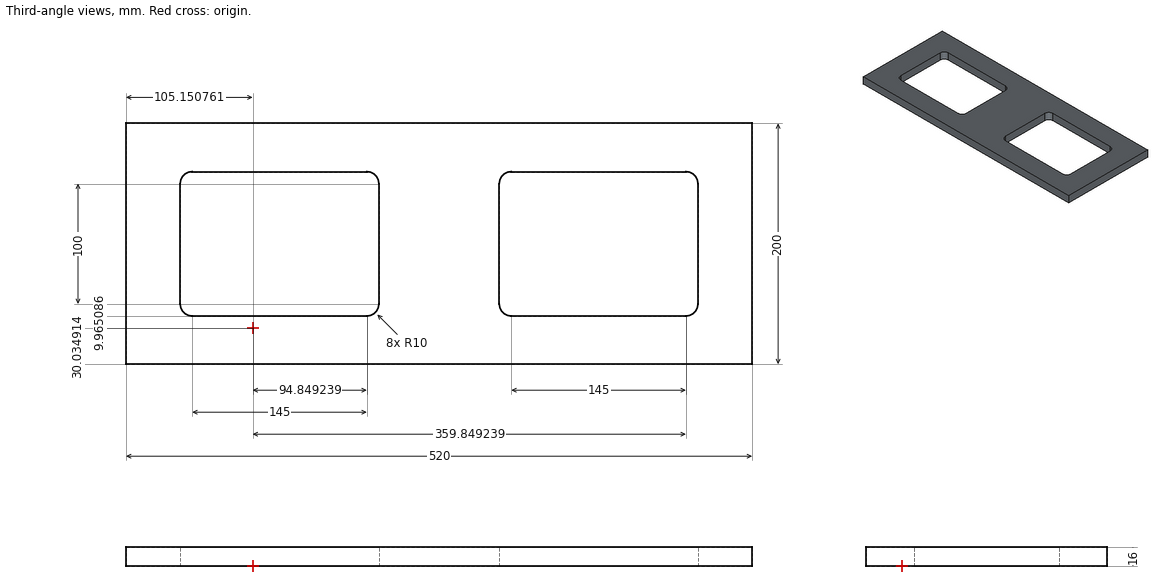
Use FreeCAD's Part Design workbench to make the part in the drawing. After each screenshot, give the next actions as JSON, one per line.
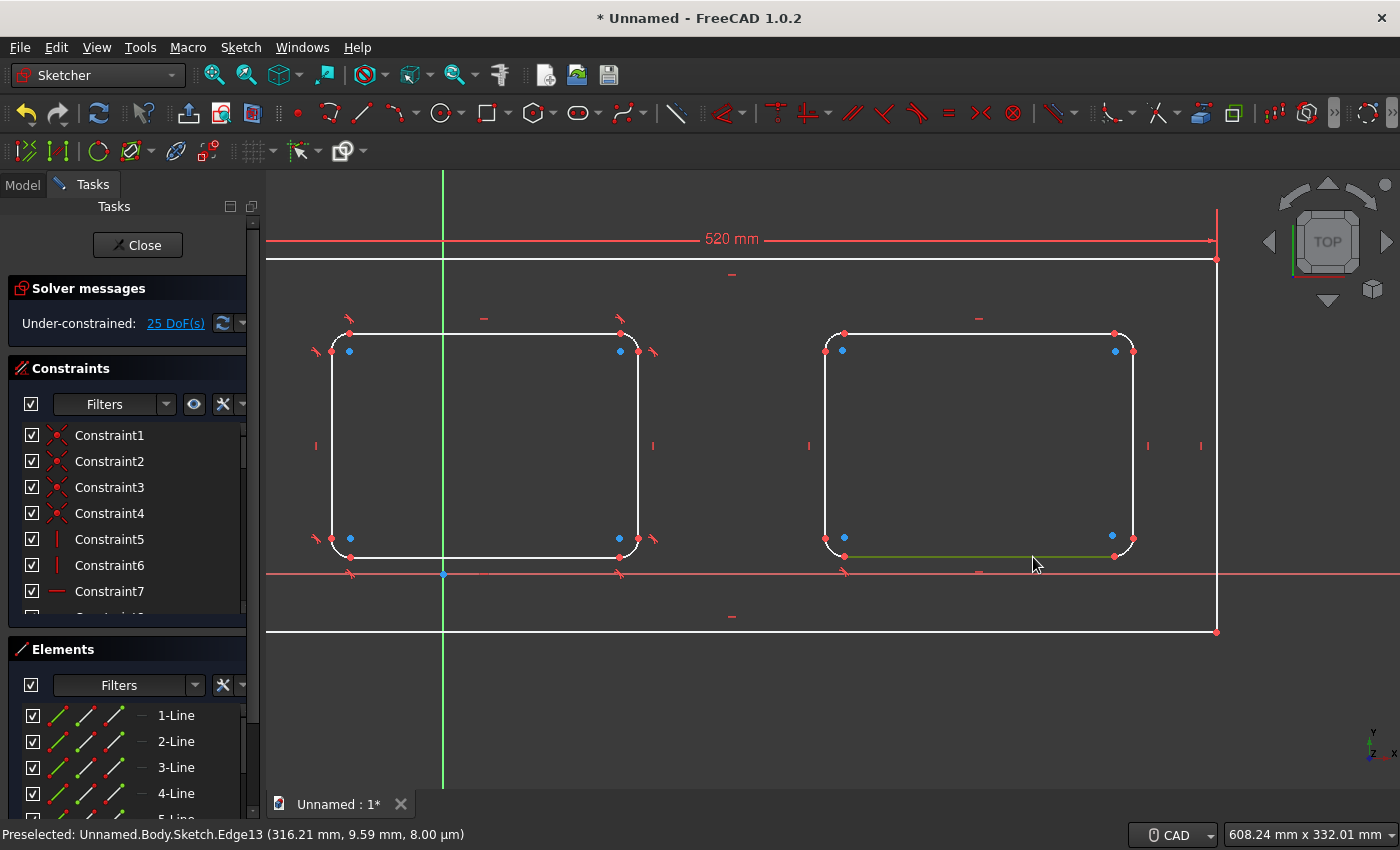
{"action": "left_click", "coordinate": [1127, 551]}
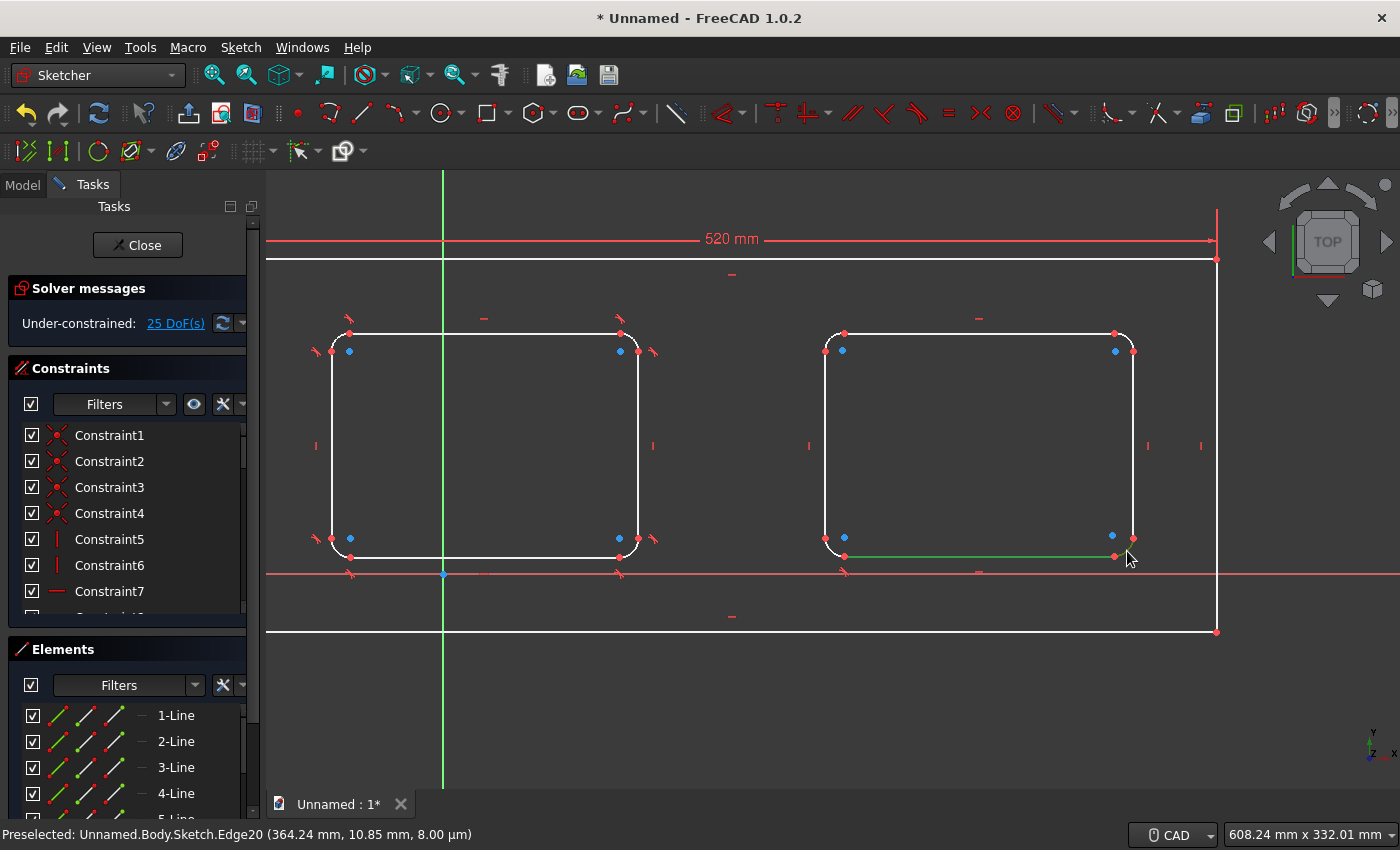
{"action": "key", "text": "t"}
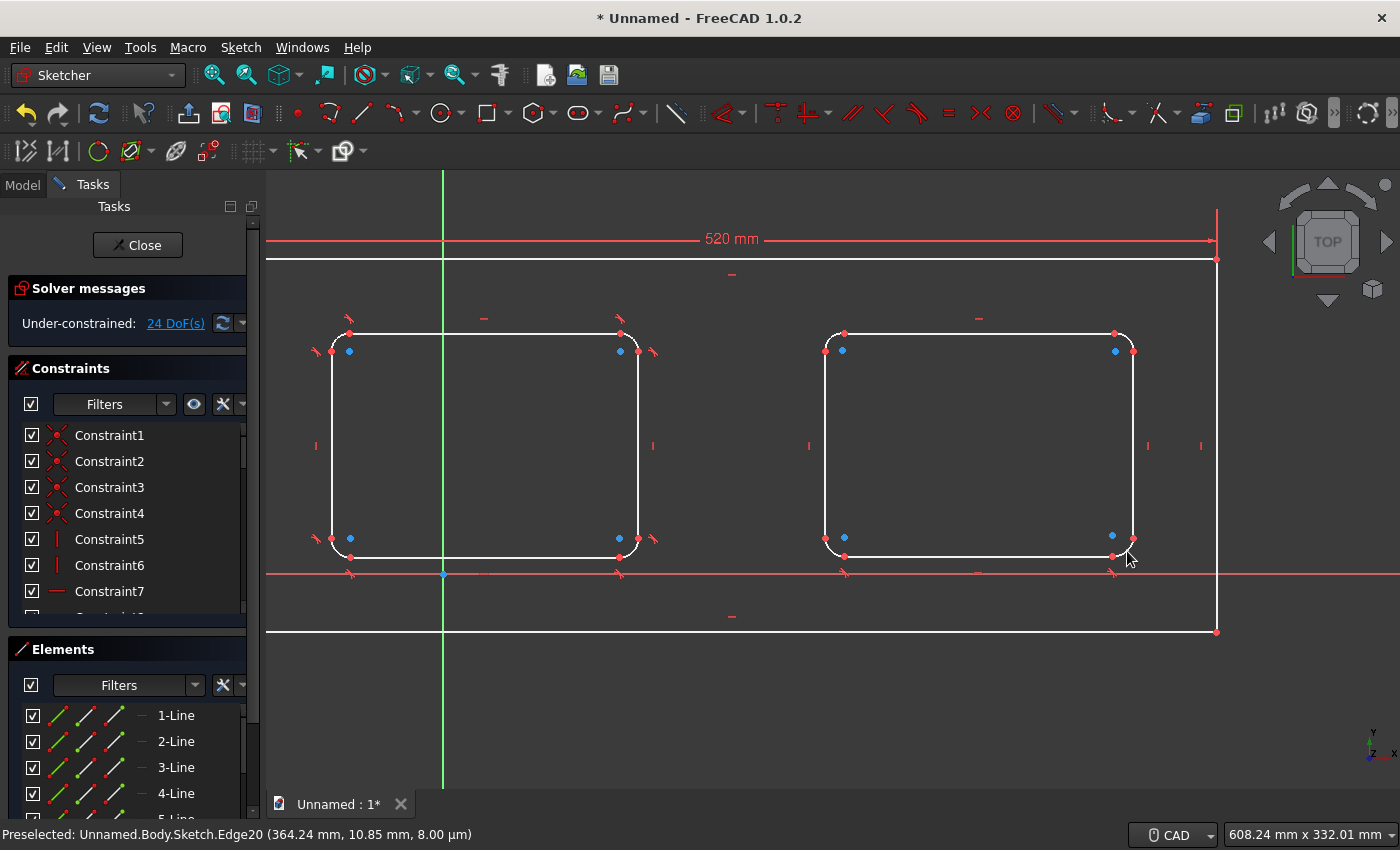
{"action": "left_click", "coordinate": [825, 482]}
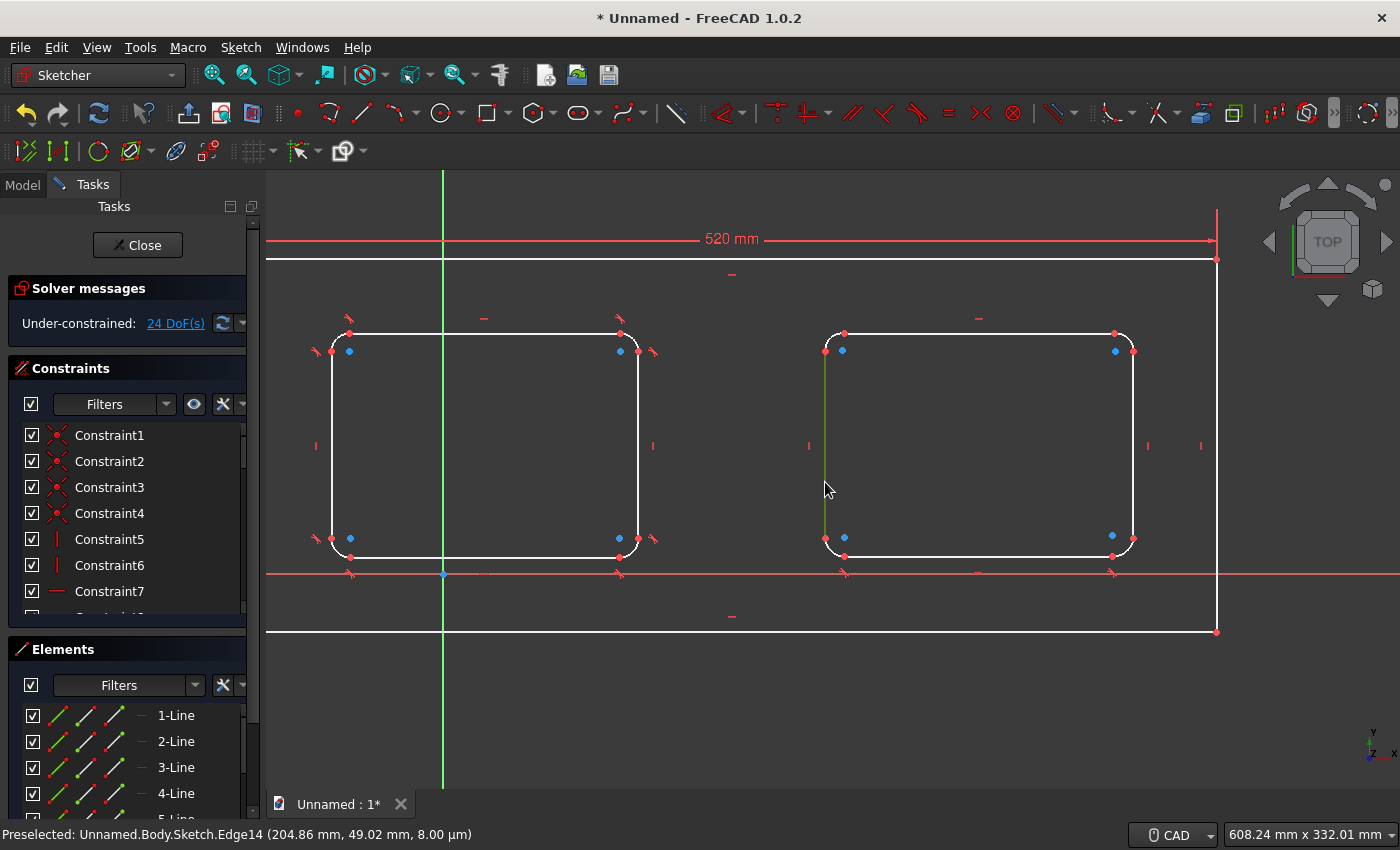
{"action": "left_click", "coordinate": [831, 551]}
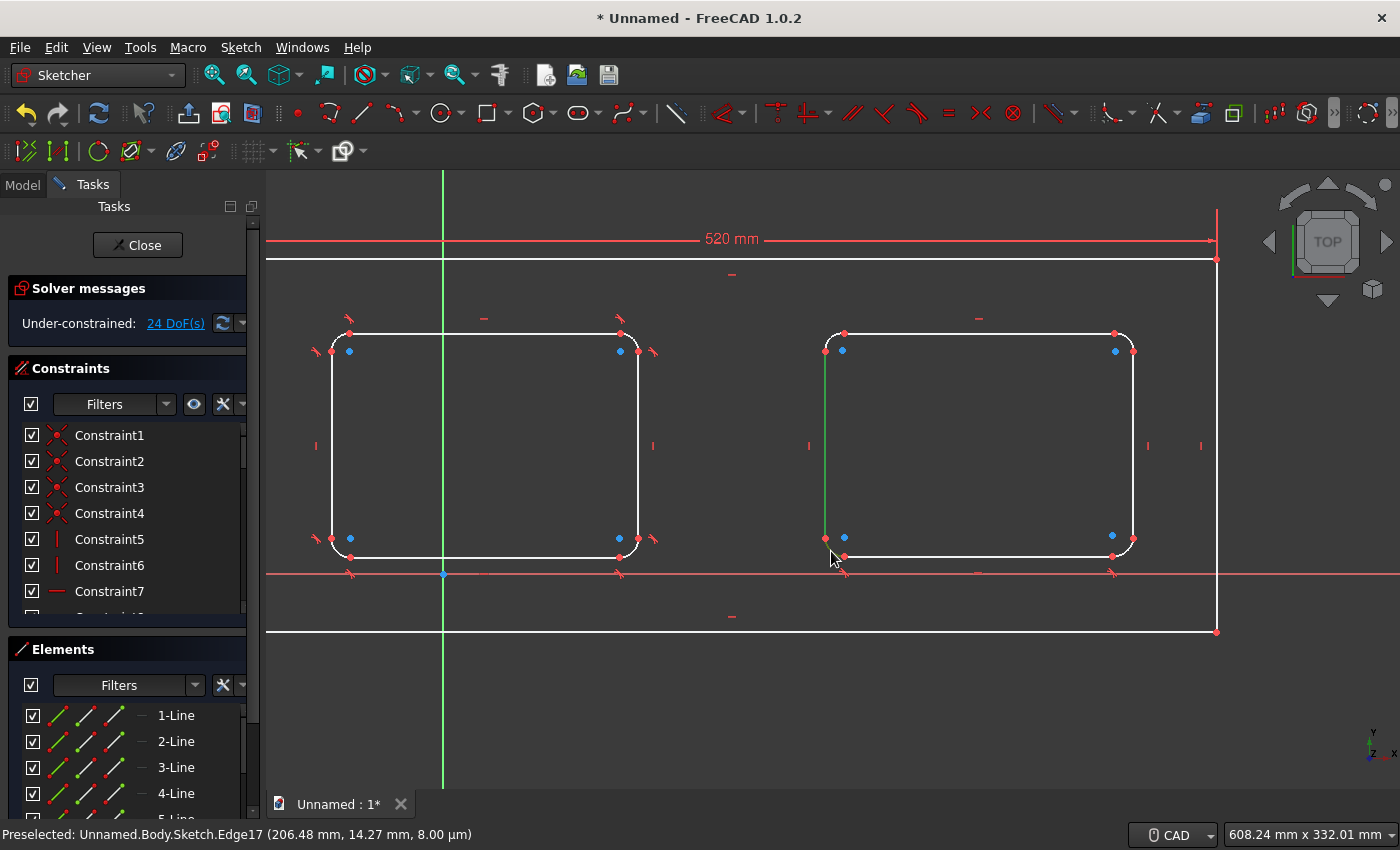
{"action": "key", "text": "t"}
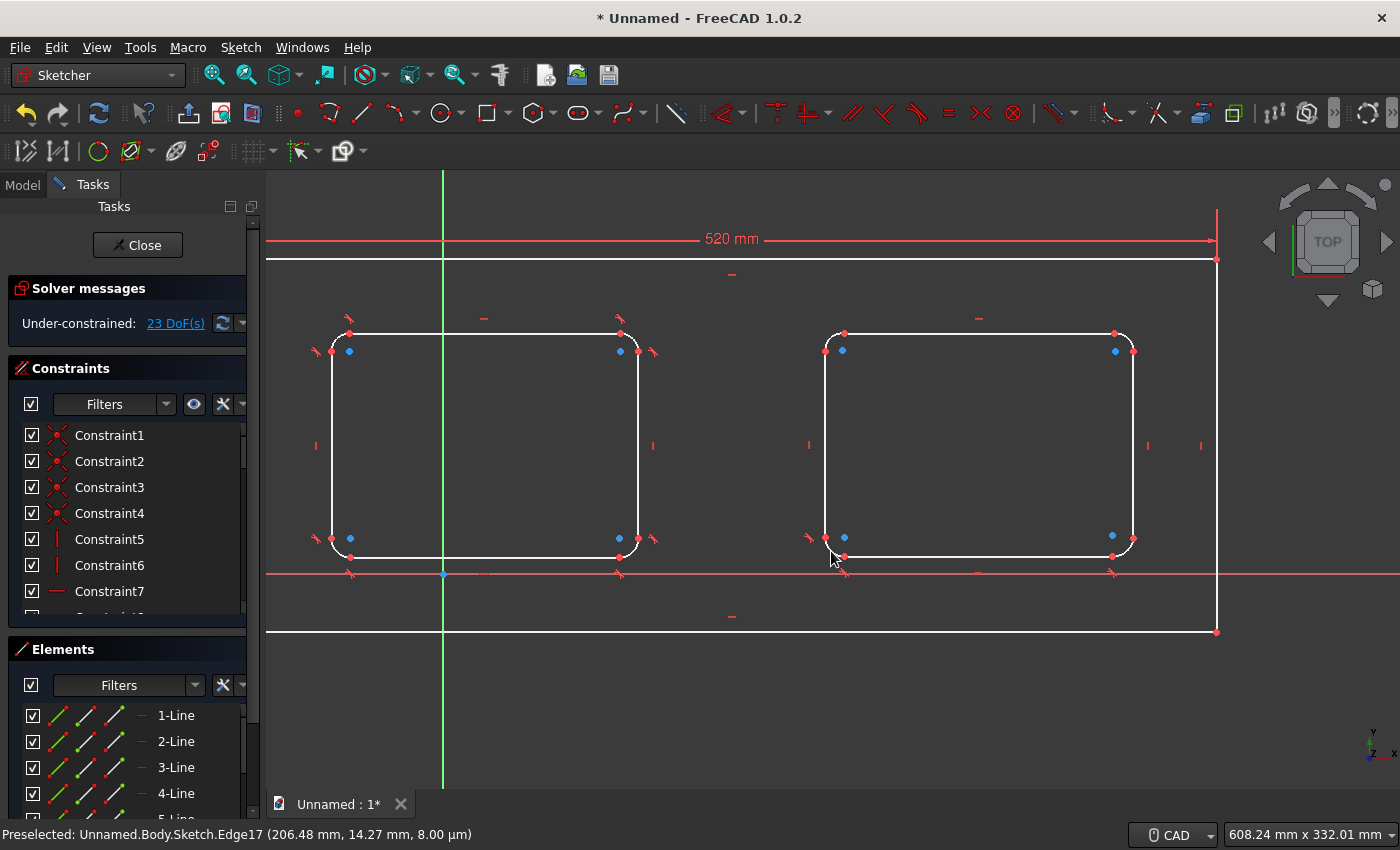
{"action": "left_click", "coordinate": [825, 482]}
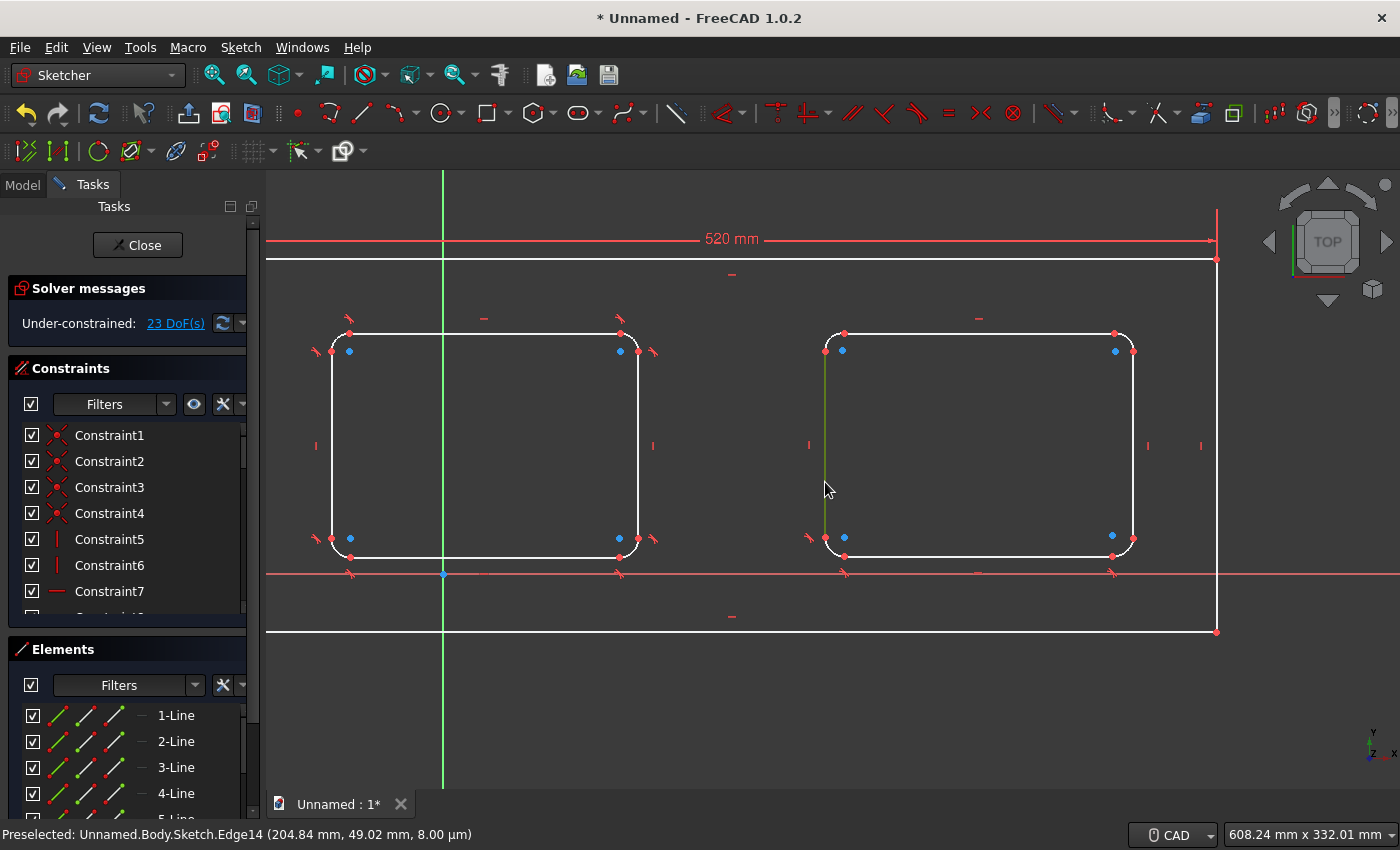
{"action": "left_click", "coordinate": [831, 338]}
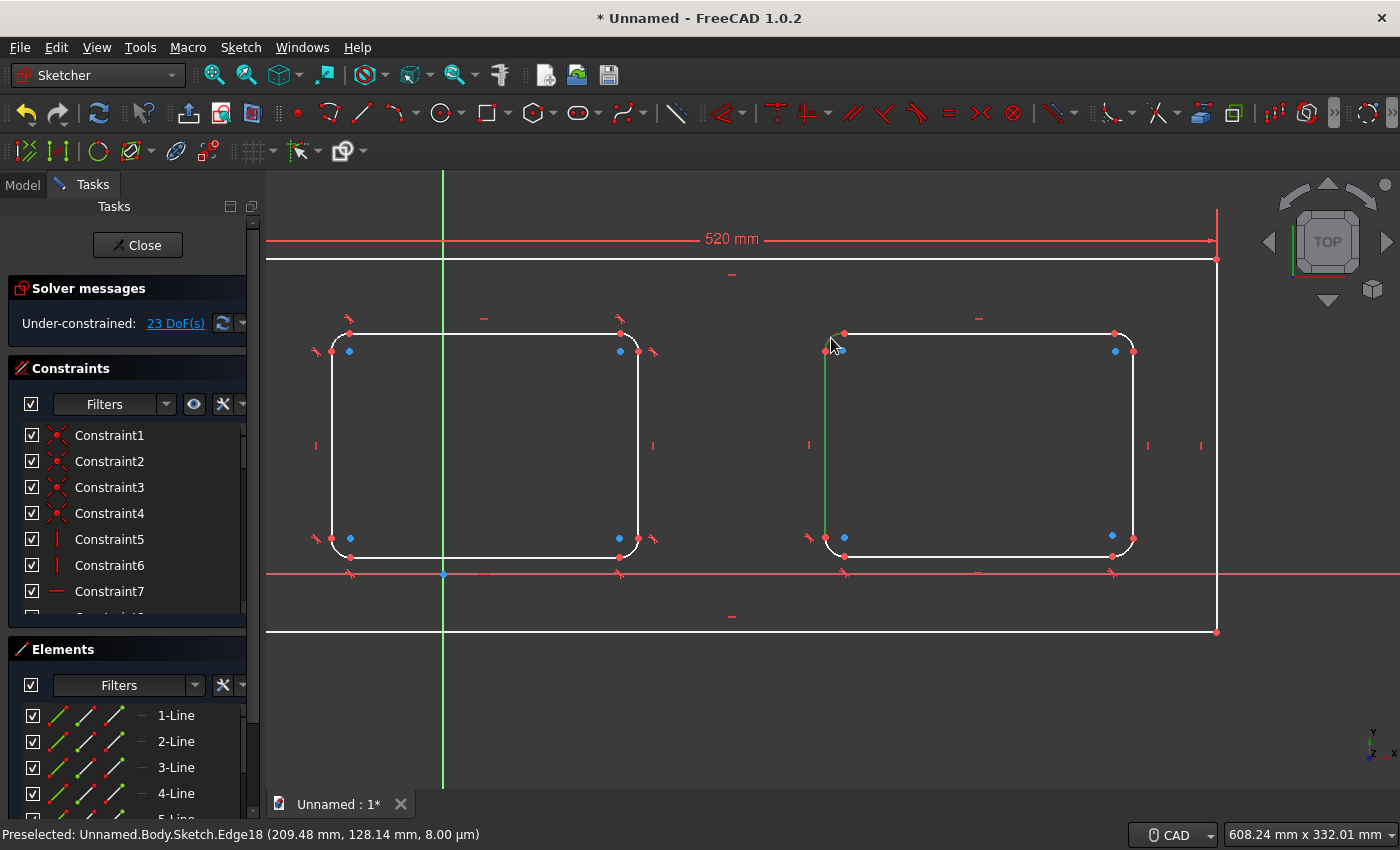
{"action": "key", "text": "t"}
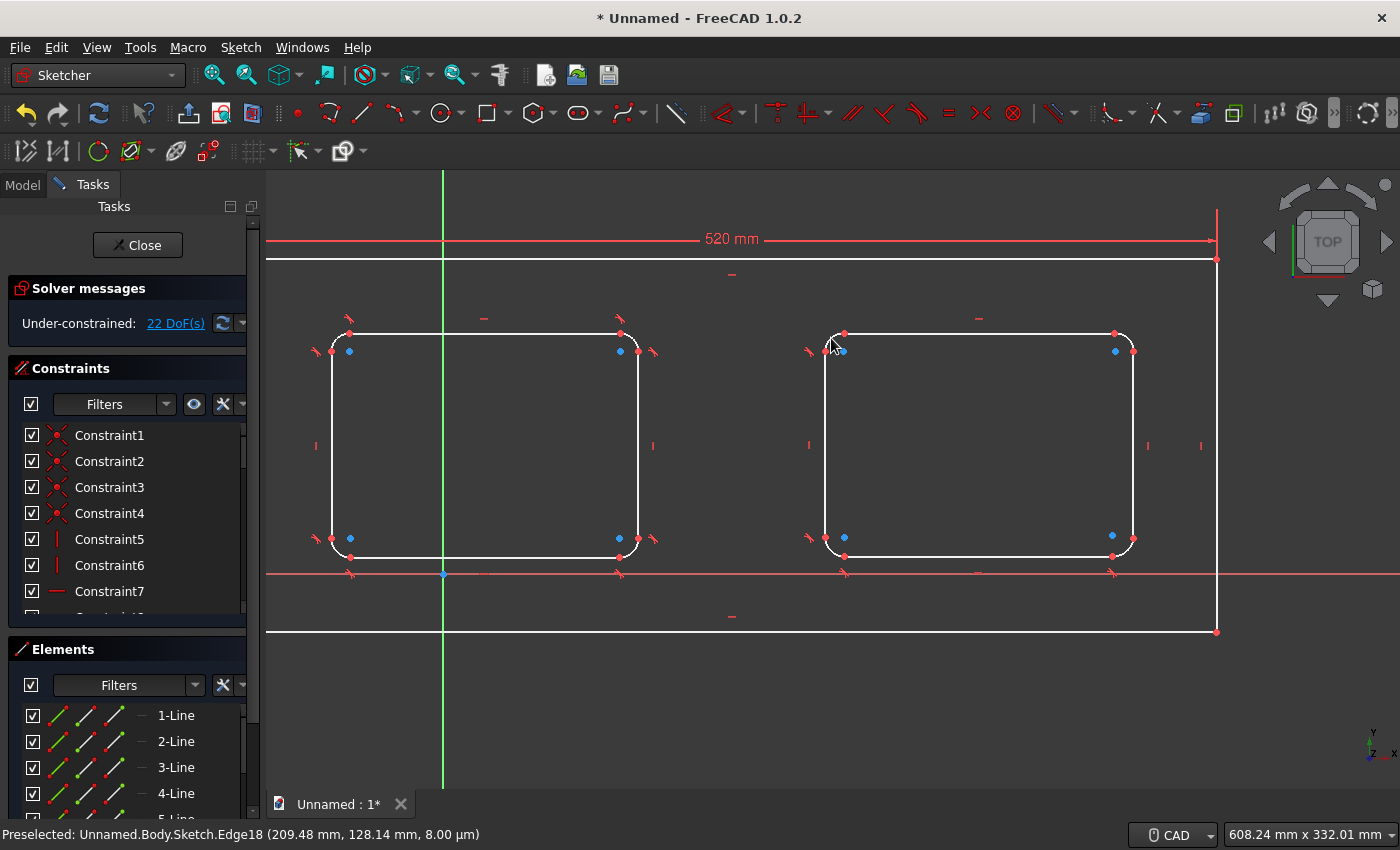
{"action": "left_click", "coordinate": [925, 334]}